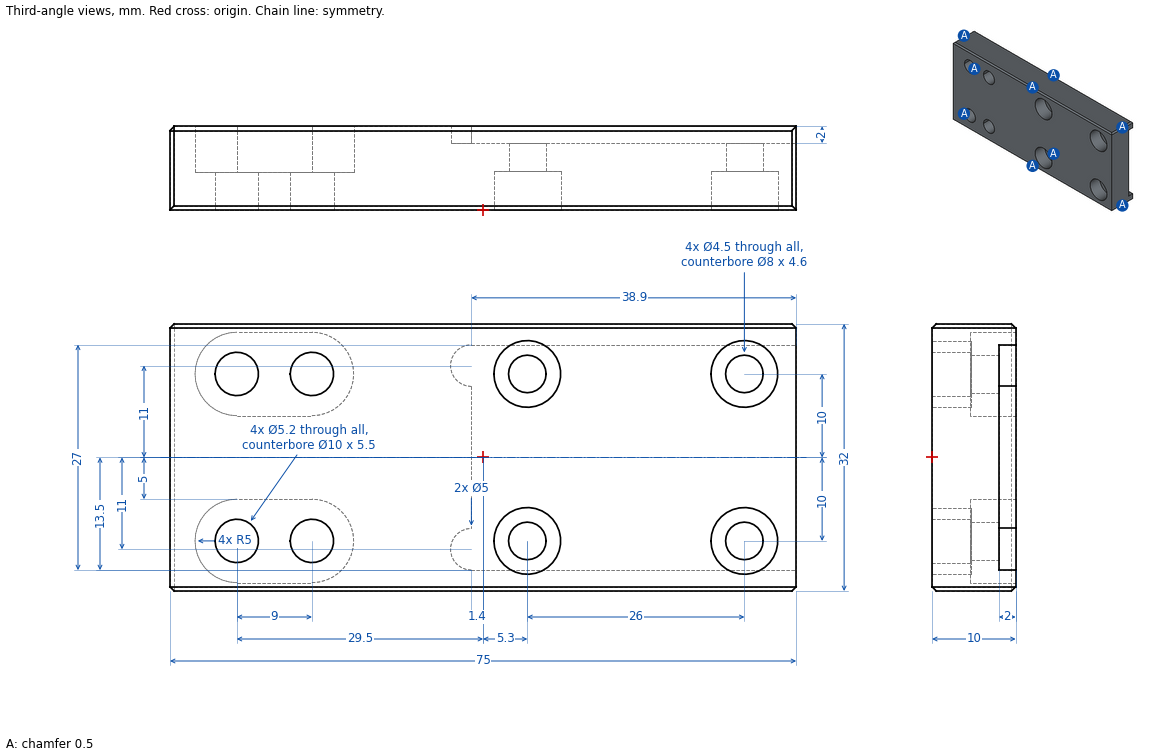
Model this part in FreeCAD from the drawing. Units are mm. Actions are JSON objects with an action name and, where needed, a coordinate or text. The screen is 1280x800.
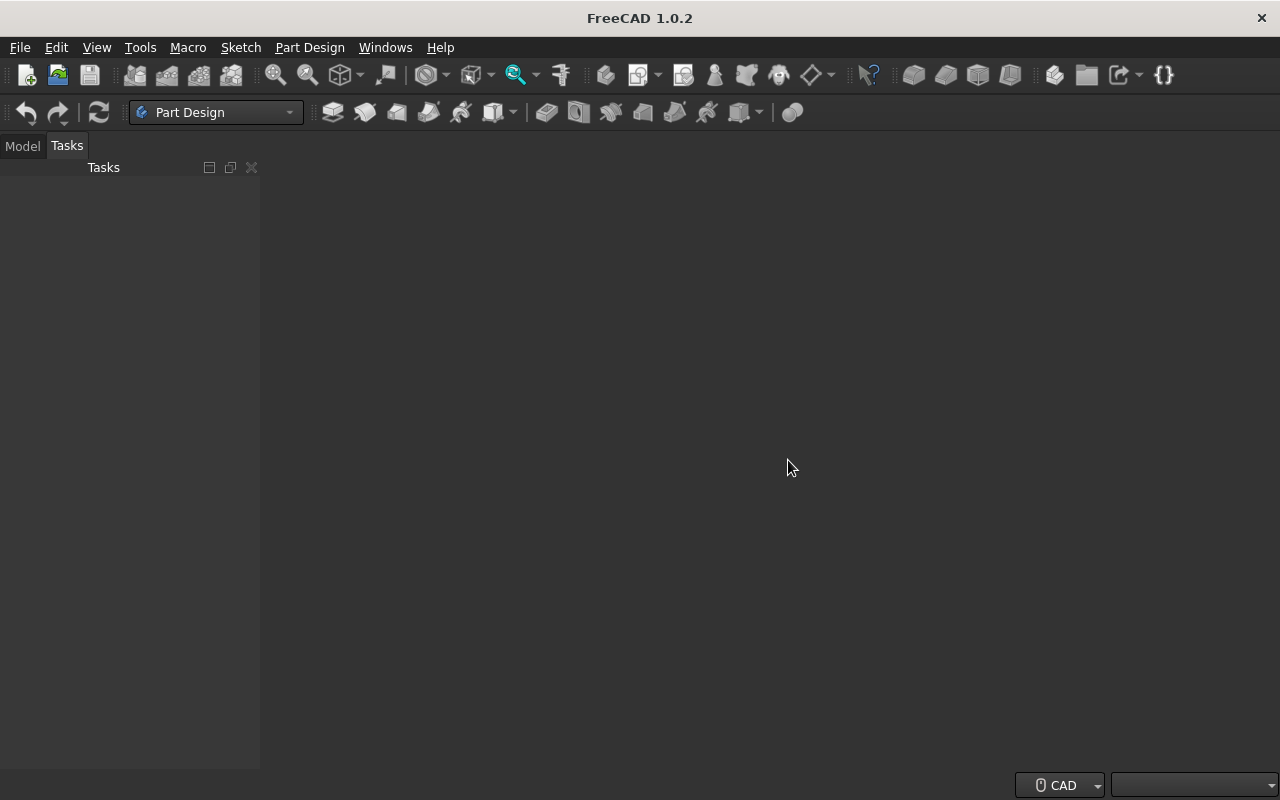
{"action": "left_click", "coordinate": [26, 76]}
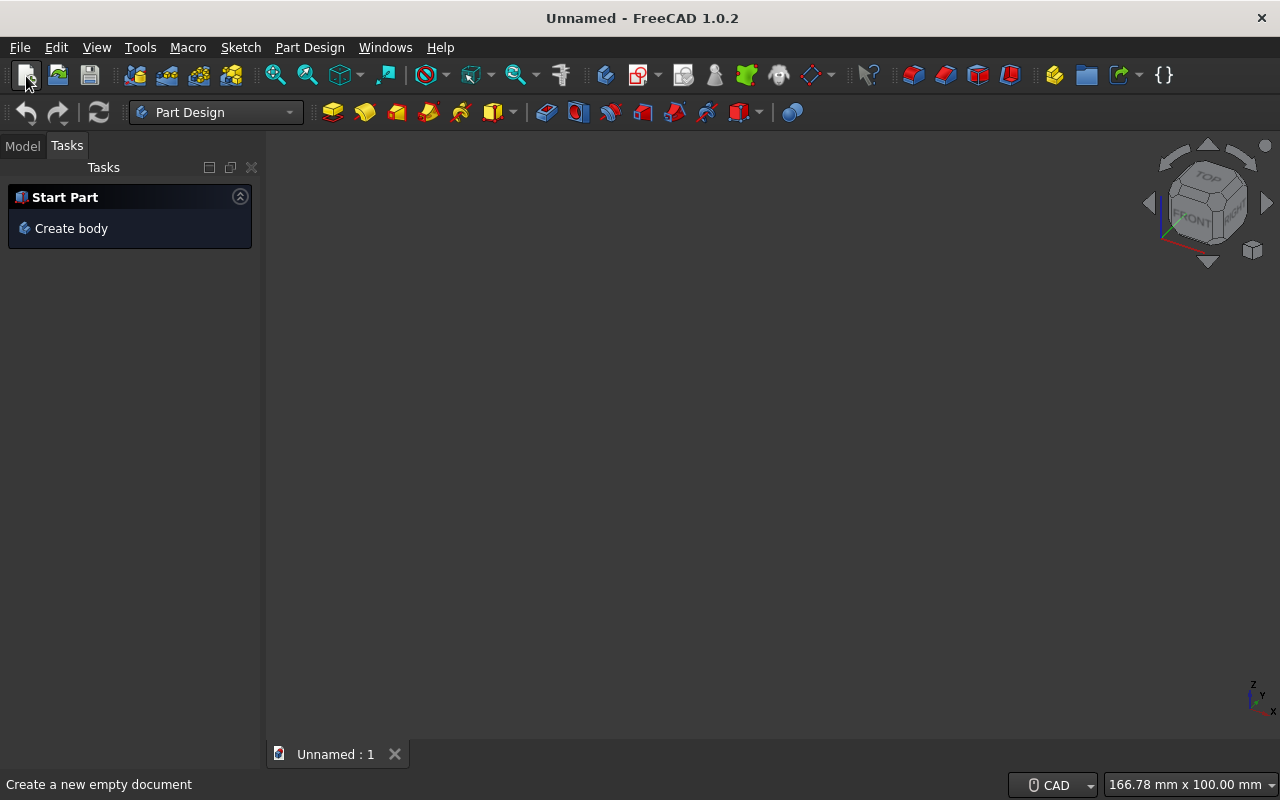
{"action": "left_click", "coordinate": [638, 76]}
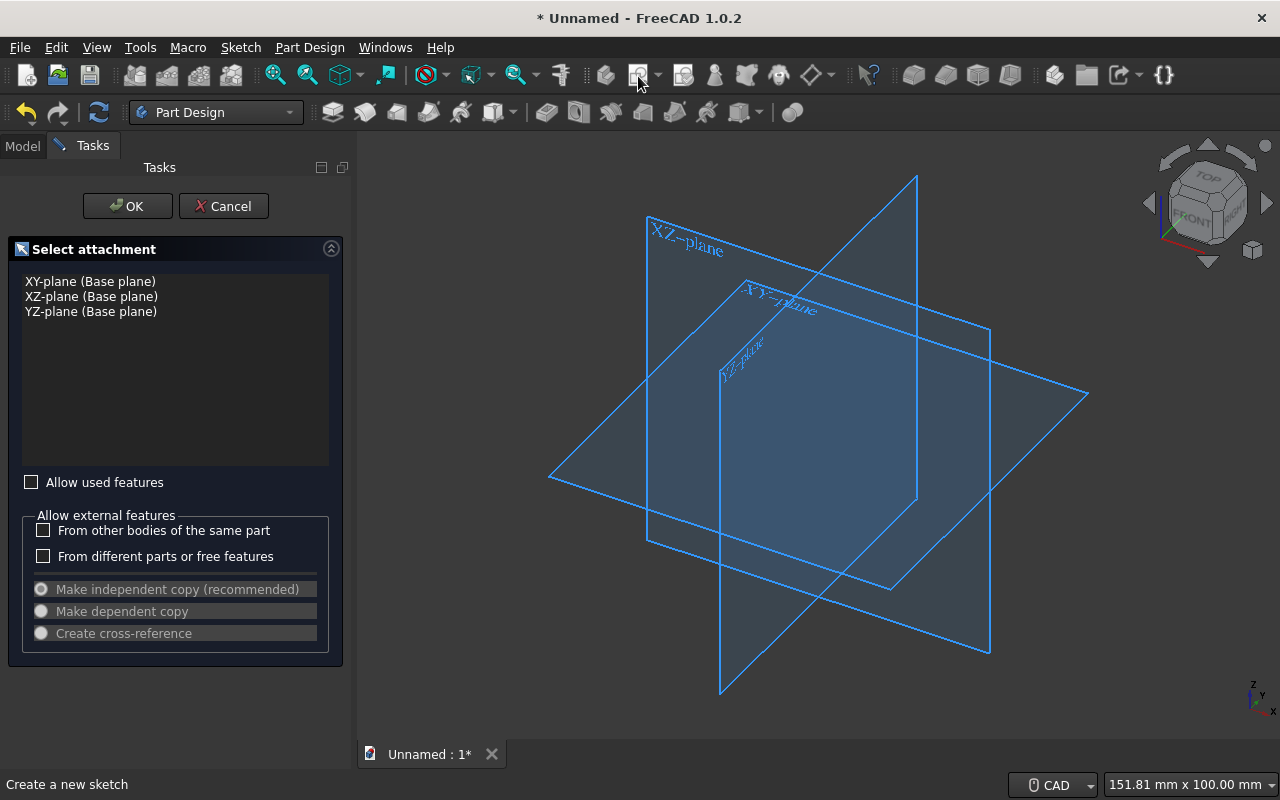
{"action": "left_click", "coordinate": [82, 296]}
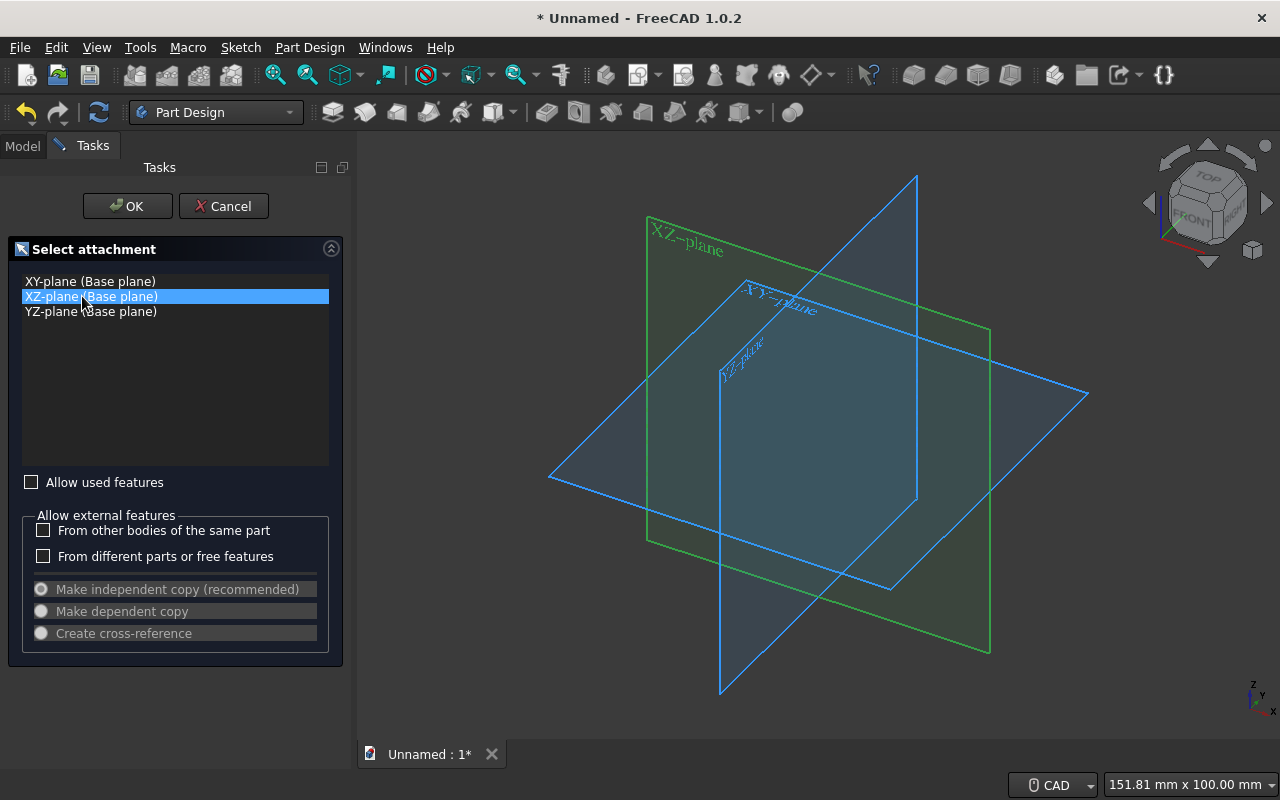
{"action": "left_click", "coordinate": [128, 206]}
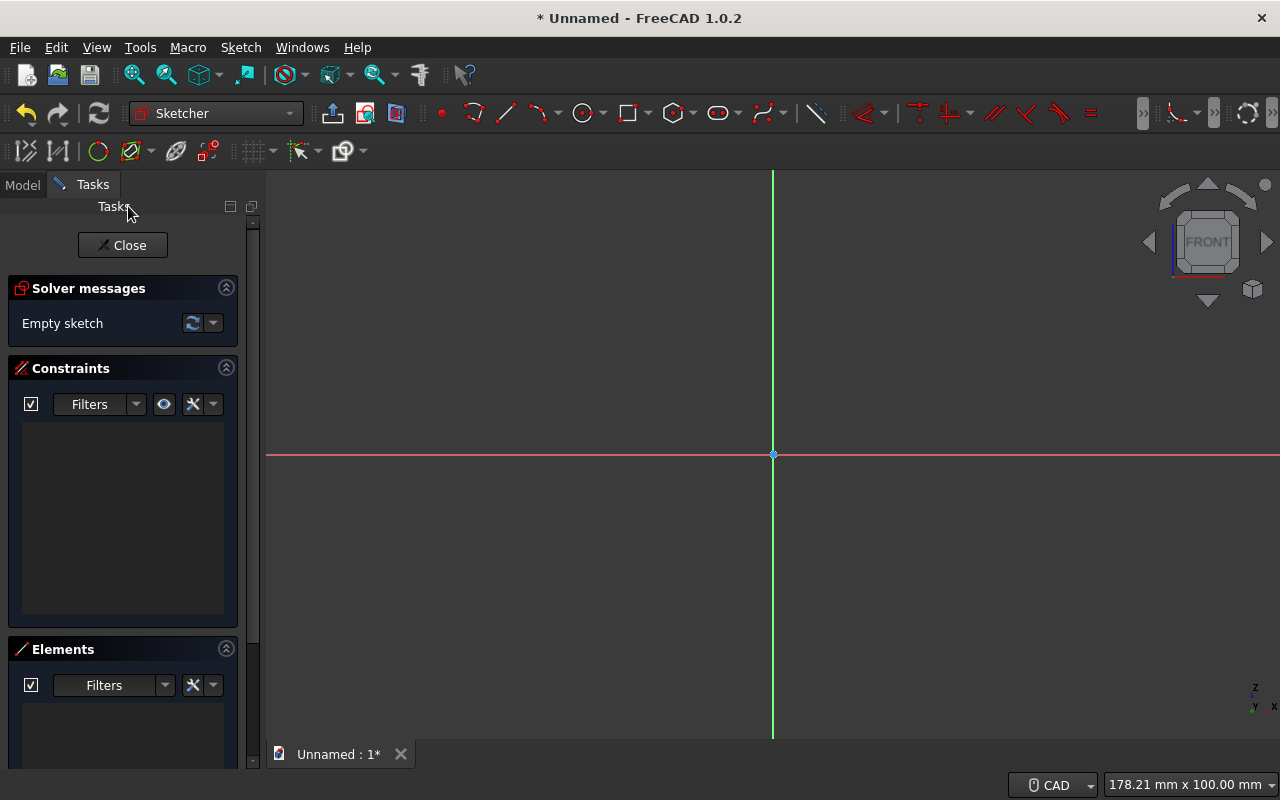
{"action": "scroll", "coordinate": [912, 455], "scroll_direction": "up", "scroll_amount": 2}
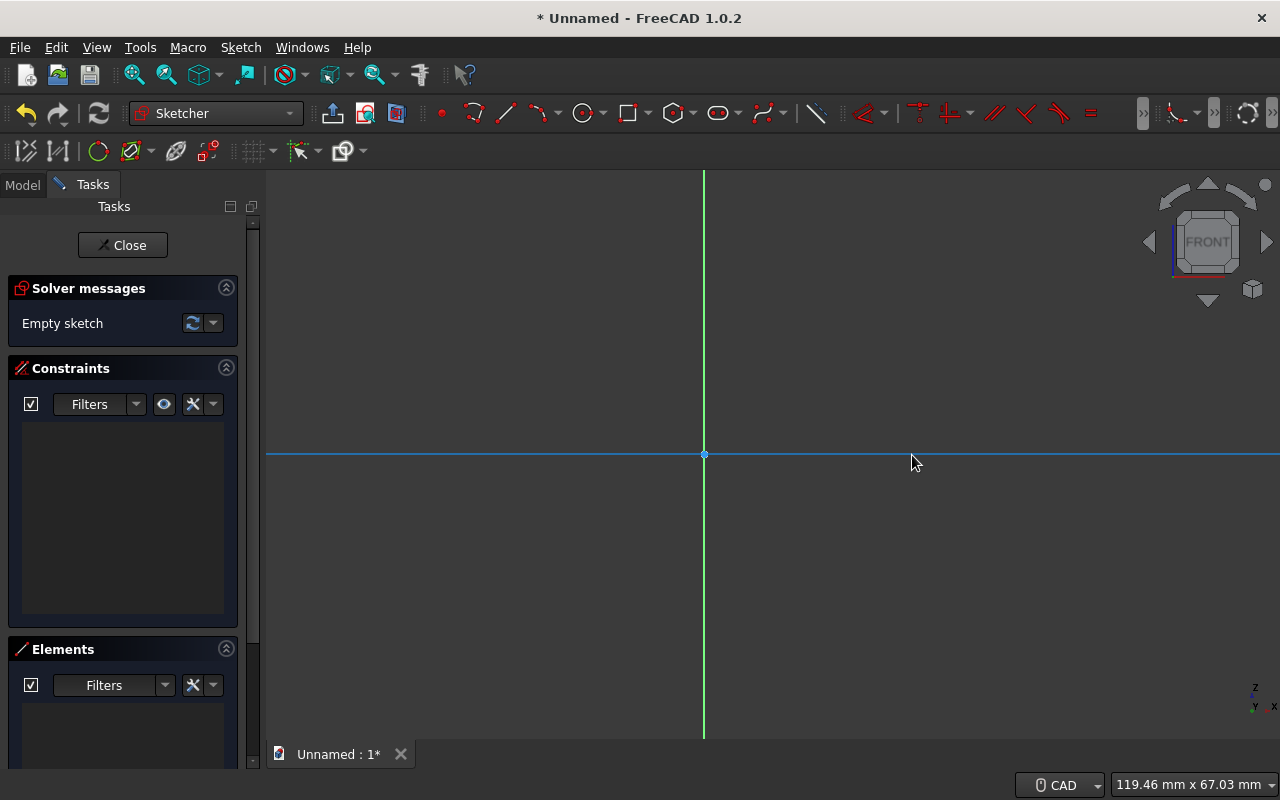
{"action": "key", "text": "g v"}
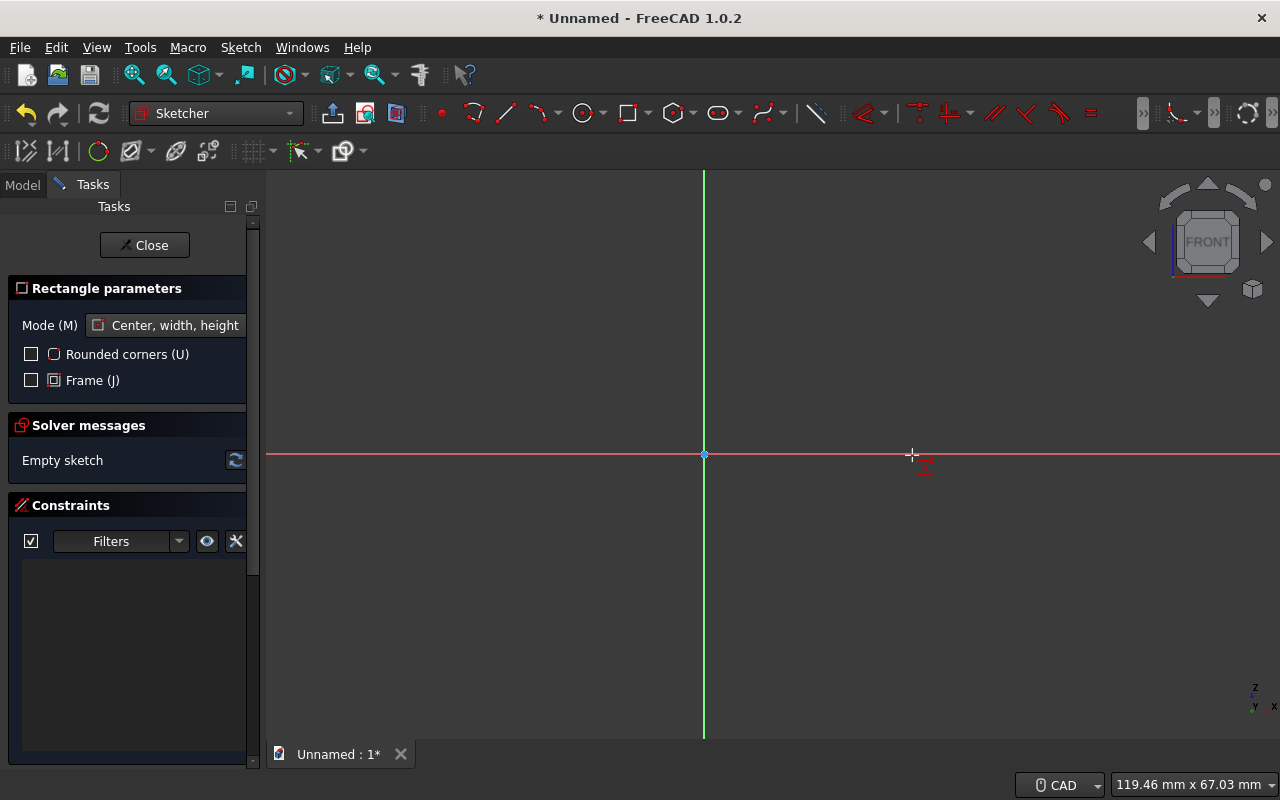
{"action": "left_click", "coordinate": [704, 454]}
{"action": "left_click", "coordinate": [1023, 318]}
{"action": "key", "text": "Escape"}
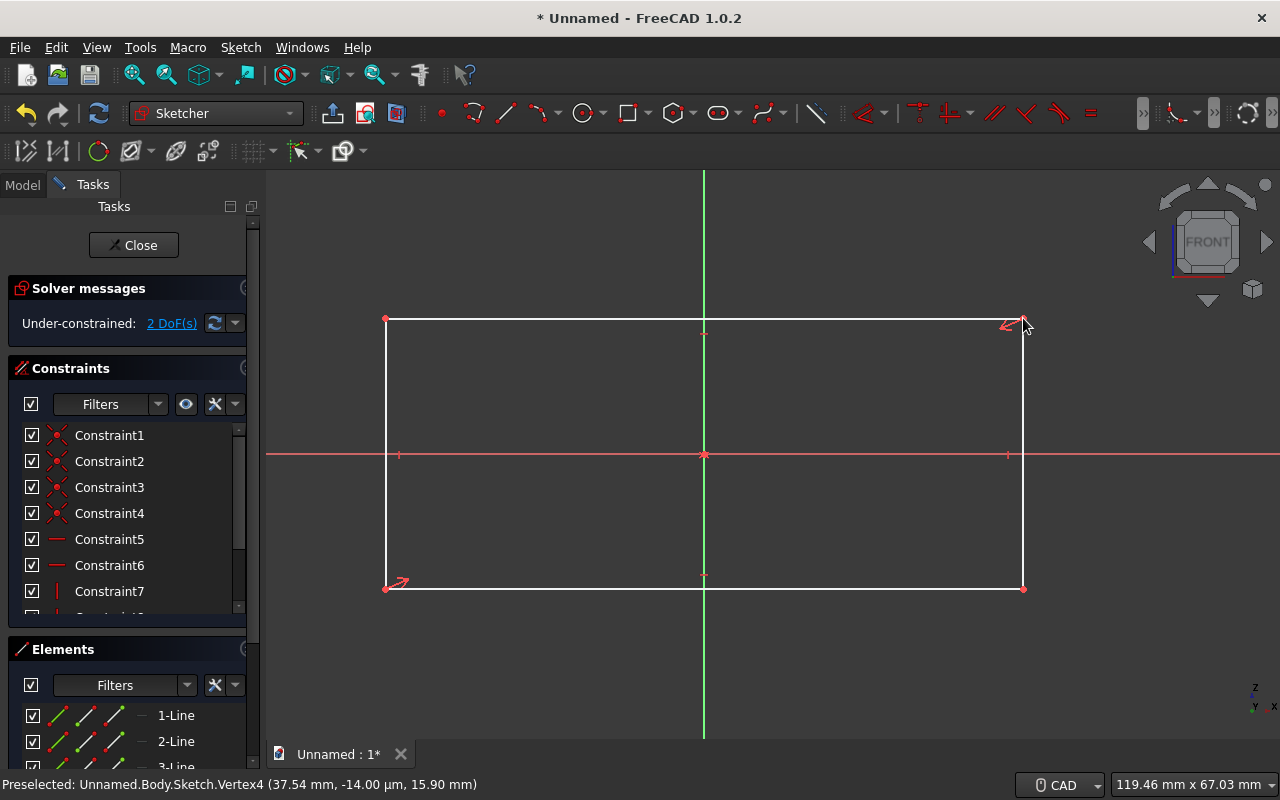
{"action": "left_click", "coordinate": [864, 114]}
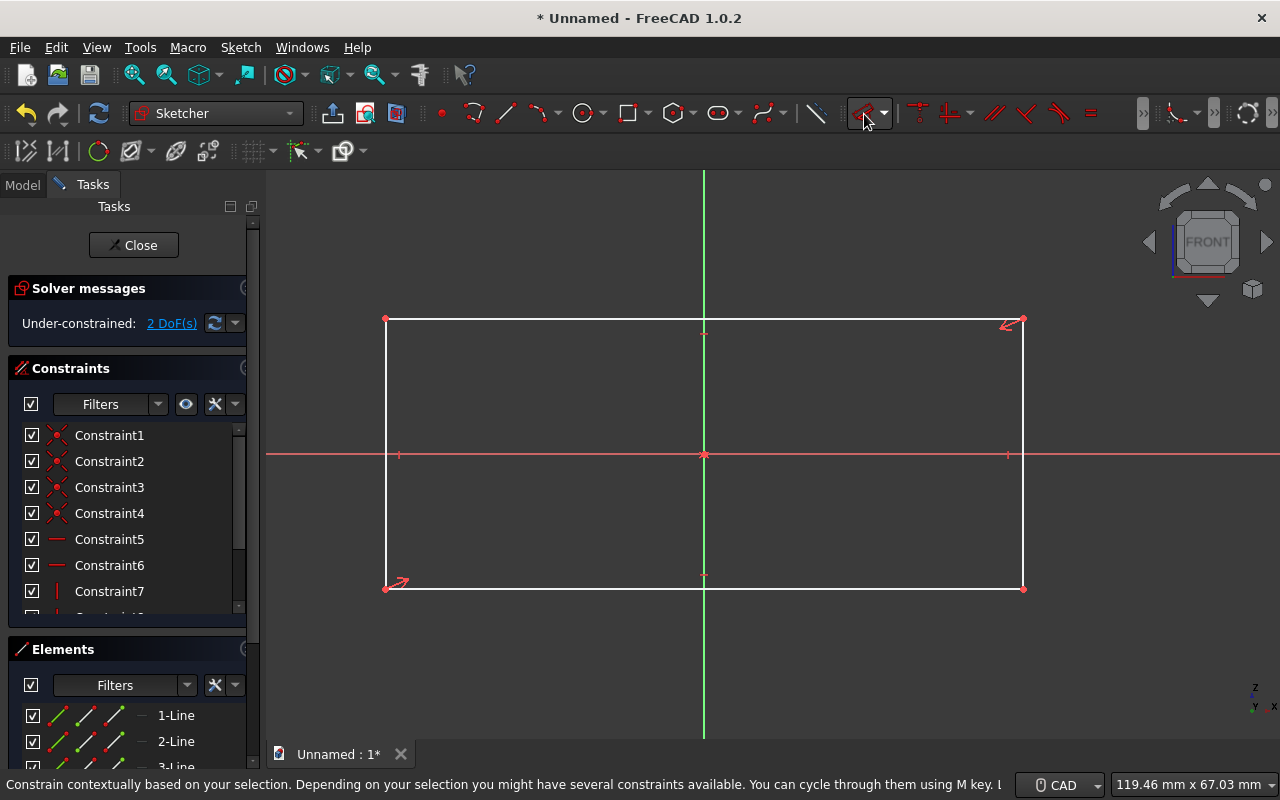
{"action": "left_click", "coordinate": [577, 589]}
{"action": "left_click", "coordinate": [558, 623]}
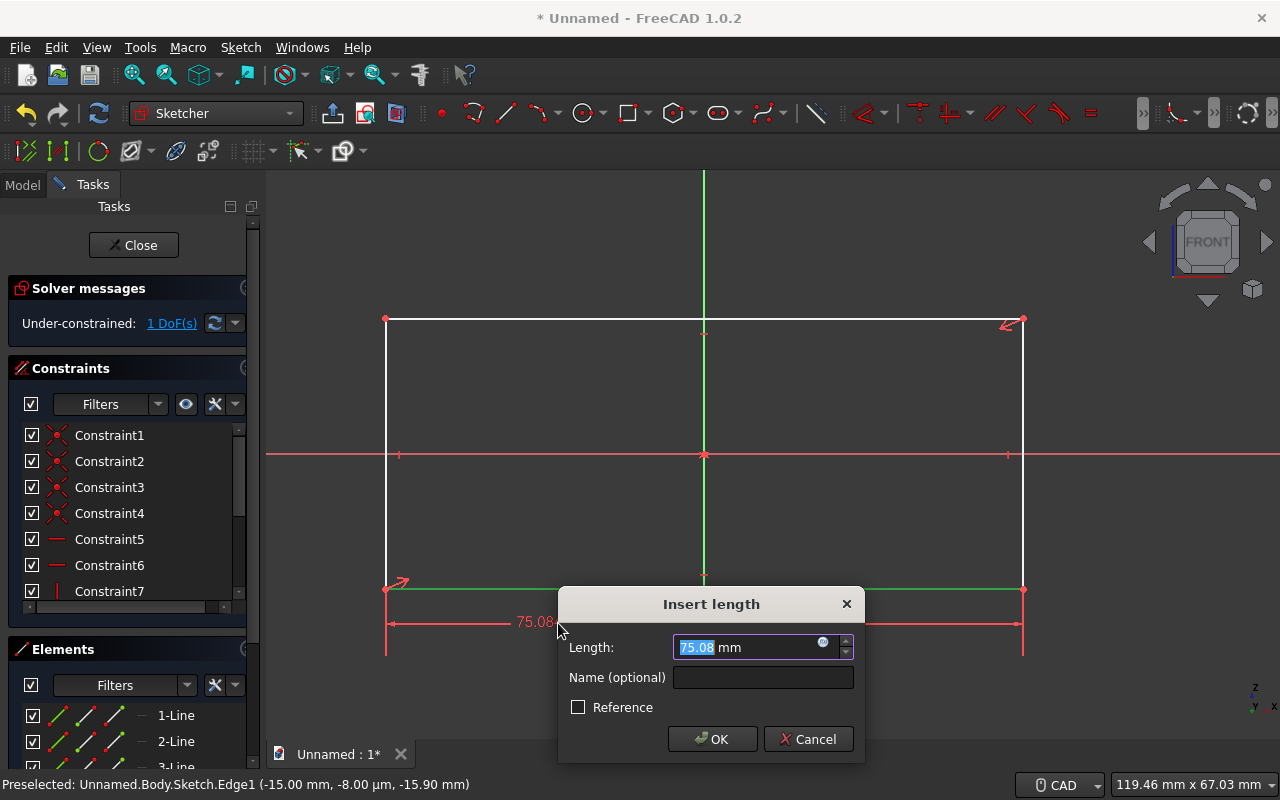
{"action": "type", "text": "75"}
{"action": "key", "text": "Return"}